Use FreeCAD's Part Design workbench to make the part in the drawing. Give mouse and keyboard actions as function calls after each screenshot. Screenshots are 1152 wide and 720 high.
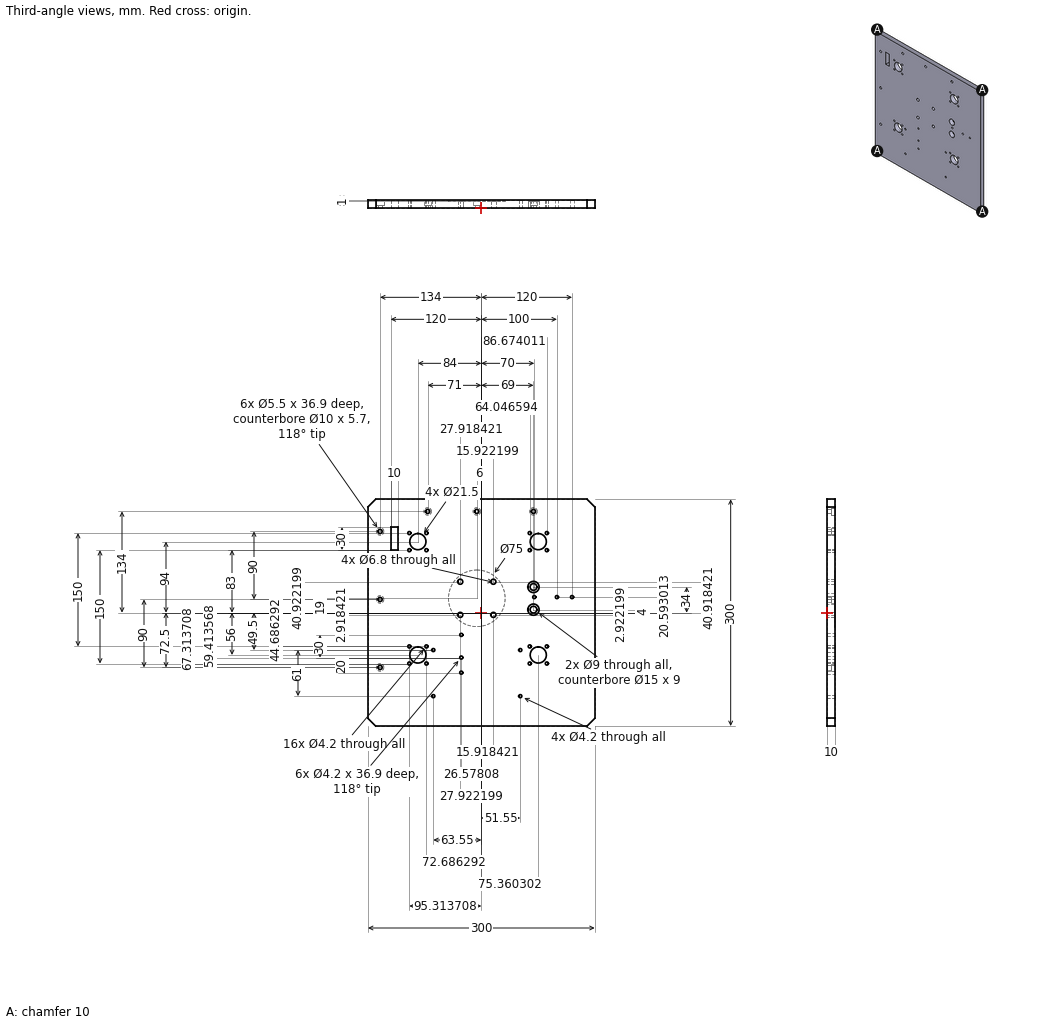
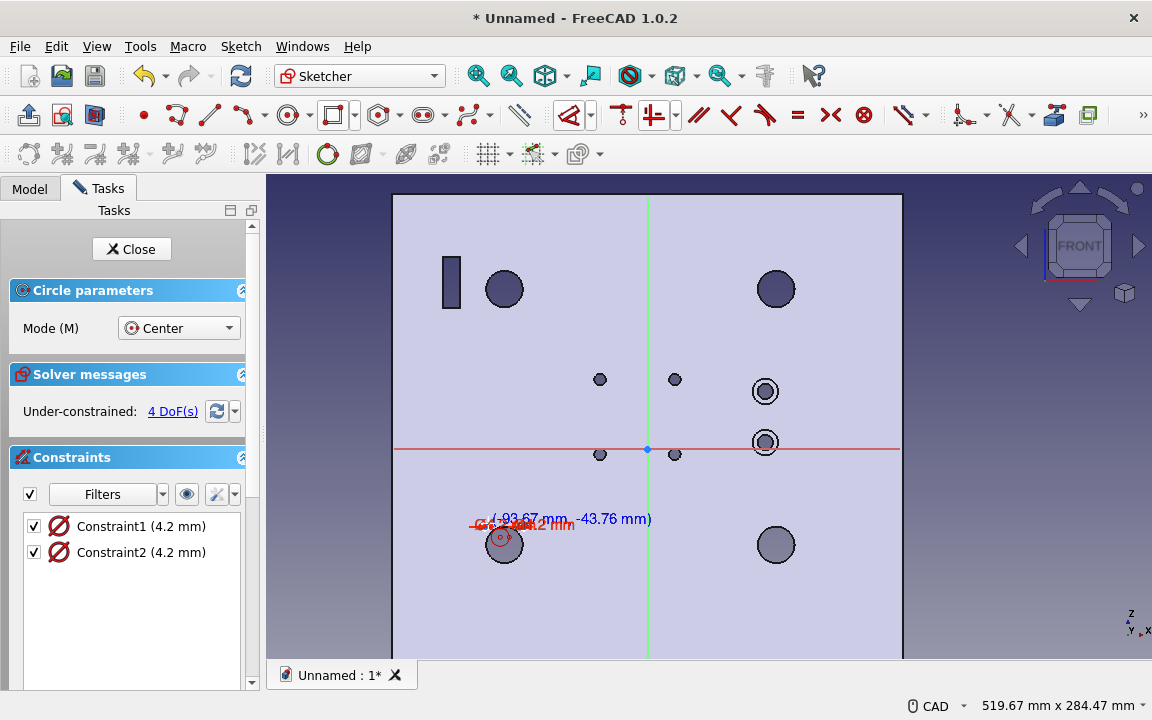
scroll(485, 564, up, 10)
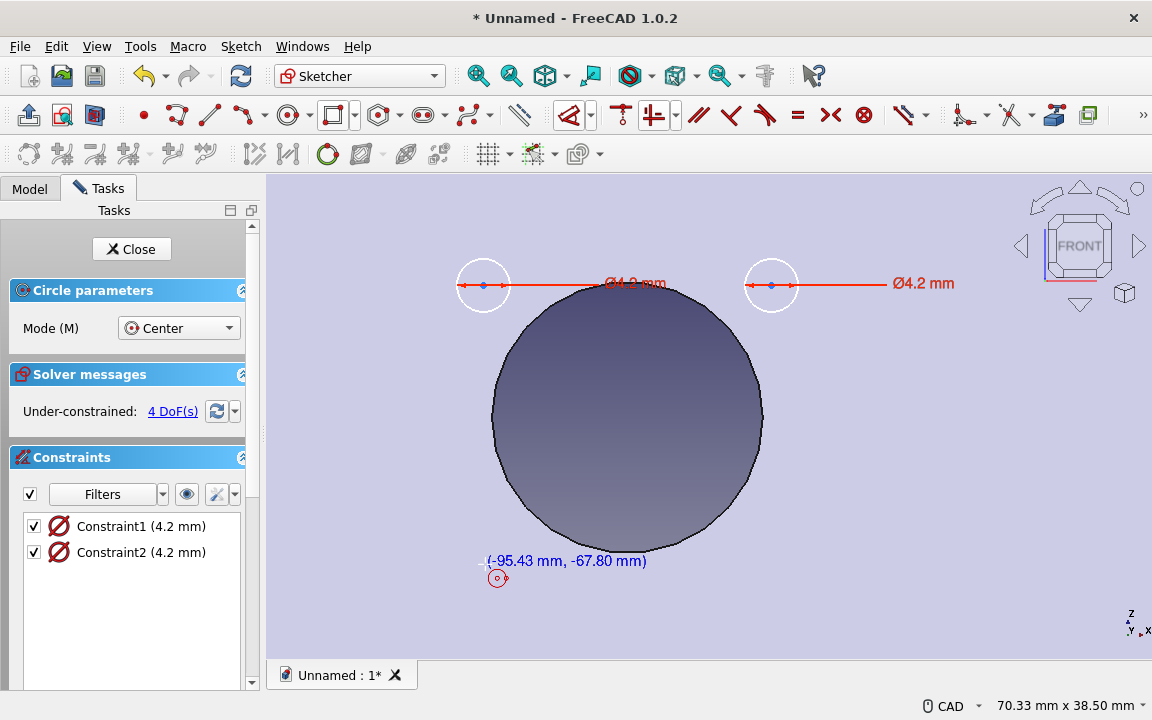
scroll(485, 564, down, 10)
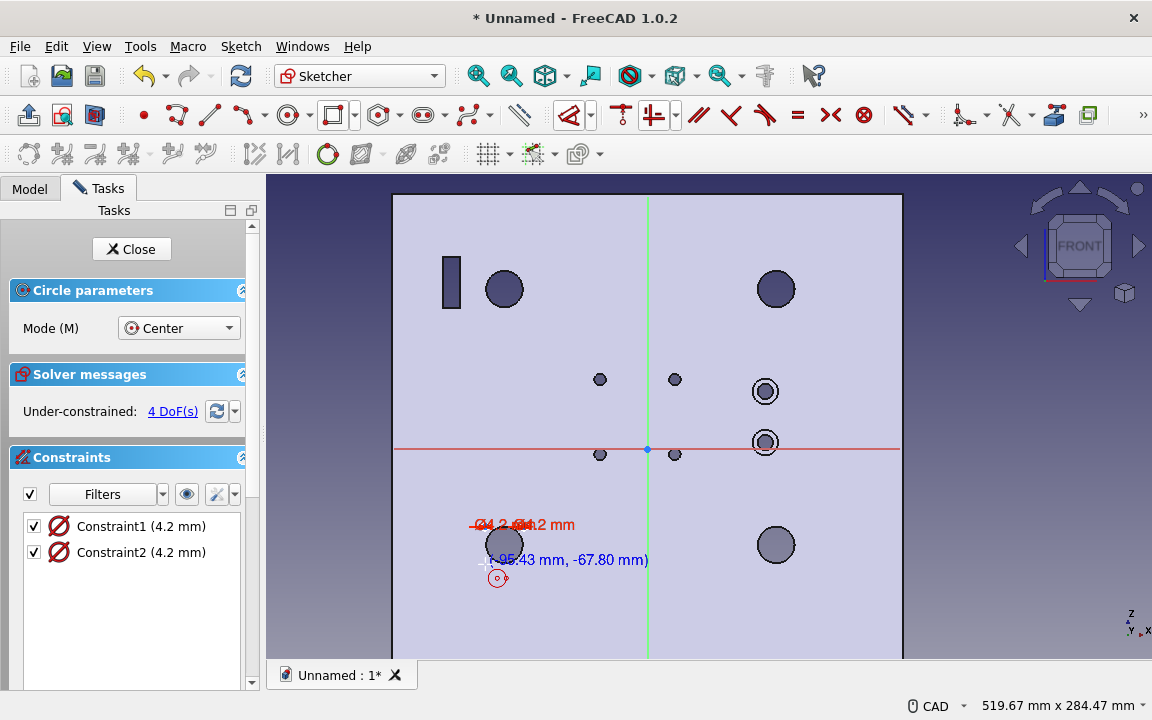
click(485, 564)
move(488, 562)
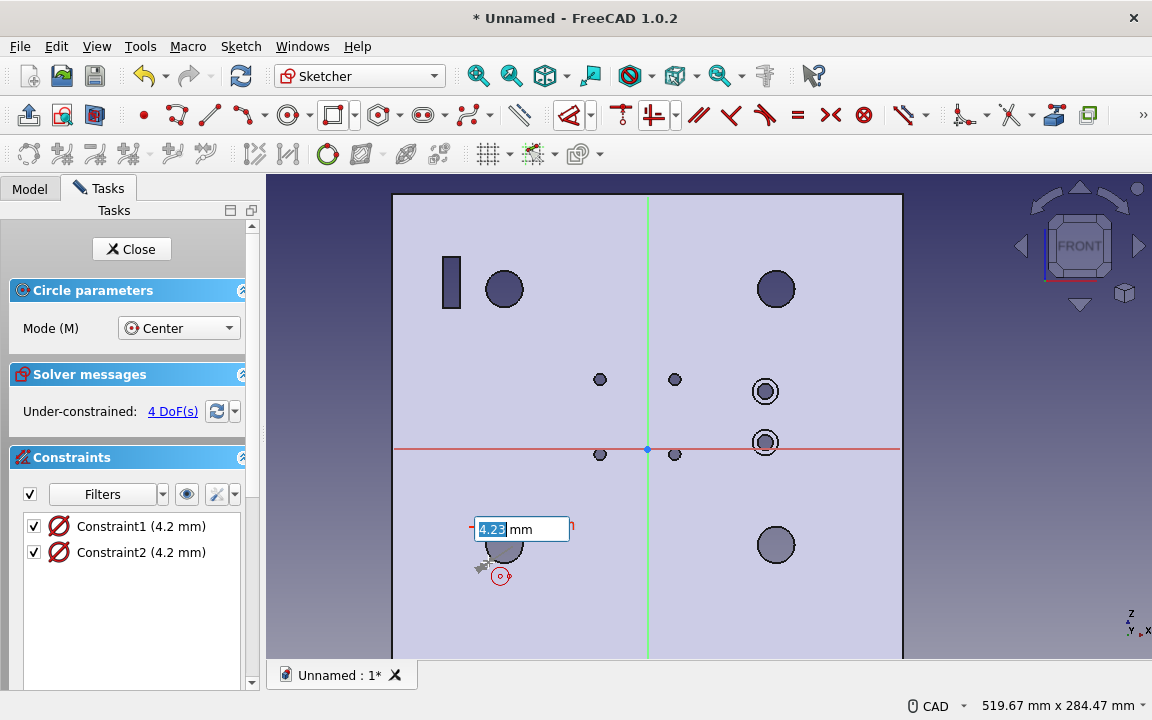
text(4.2)
key(Return)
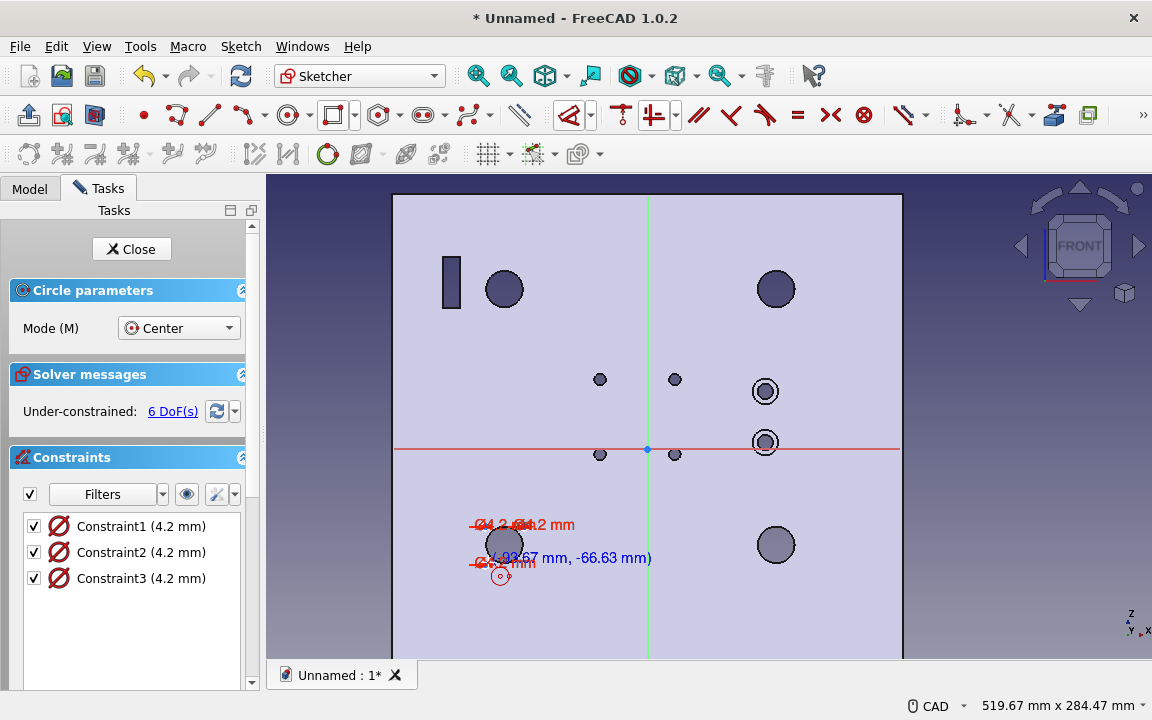
scroll(524, 564, up, 10)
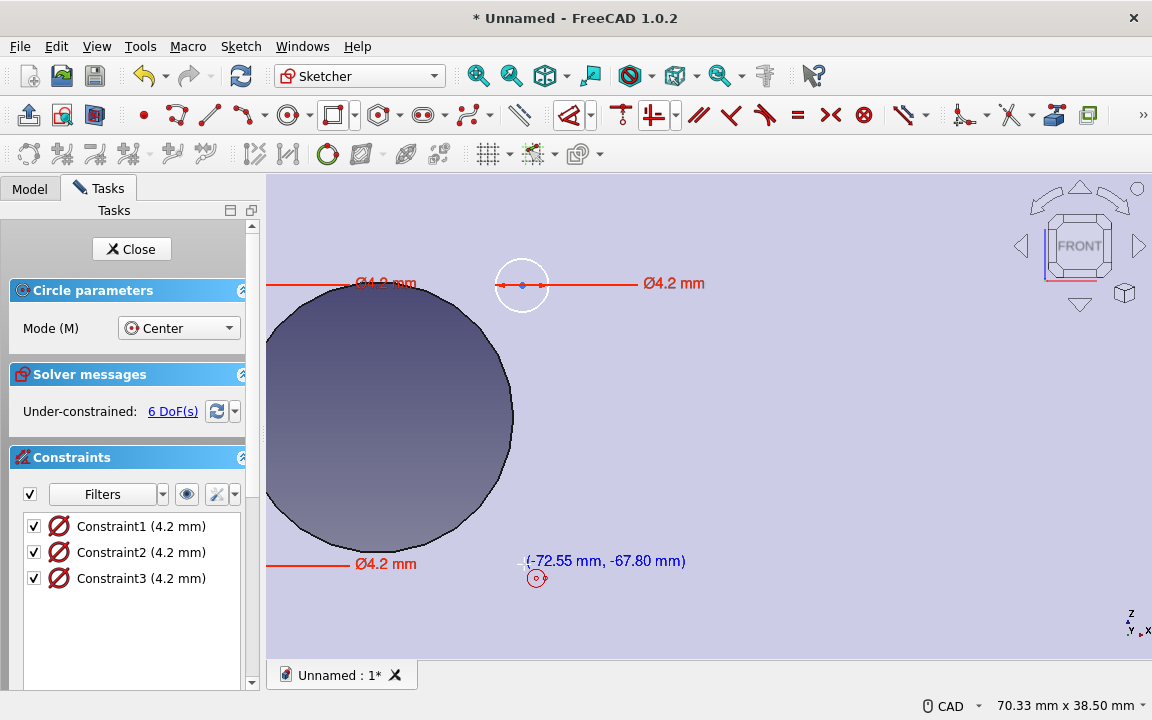
scroll(524, 564, down, 10)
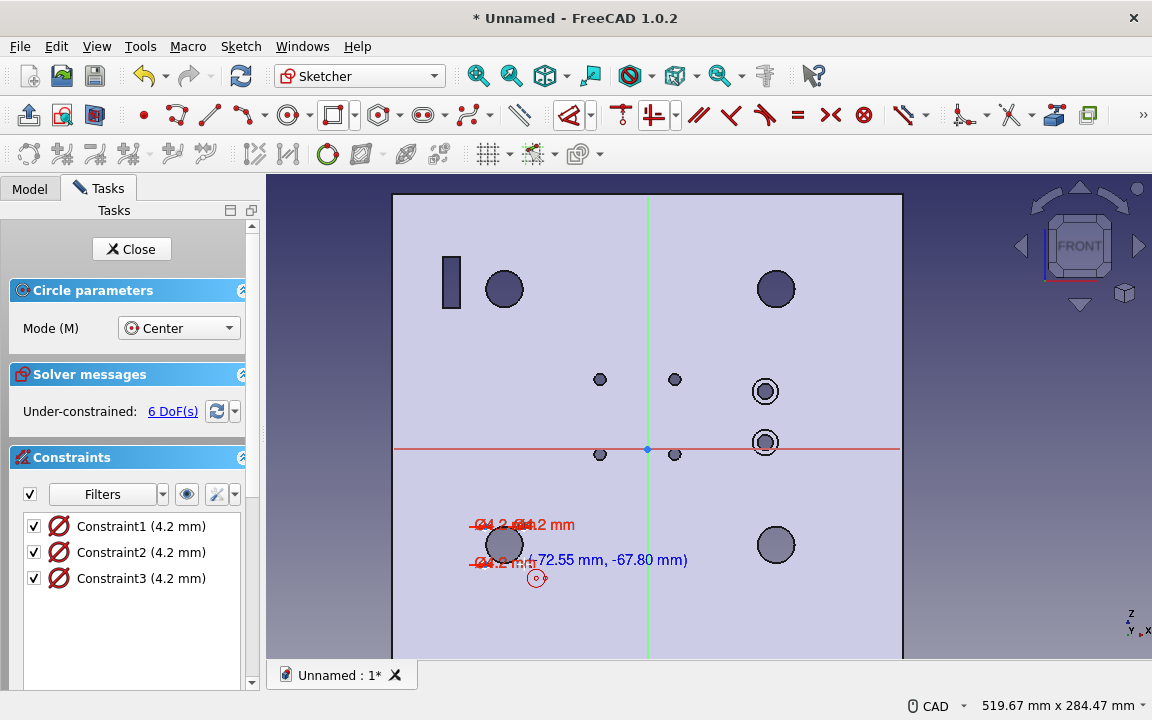
click(524, 564)
move(526, 562)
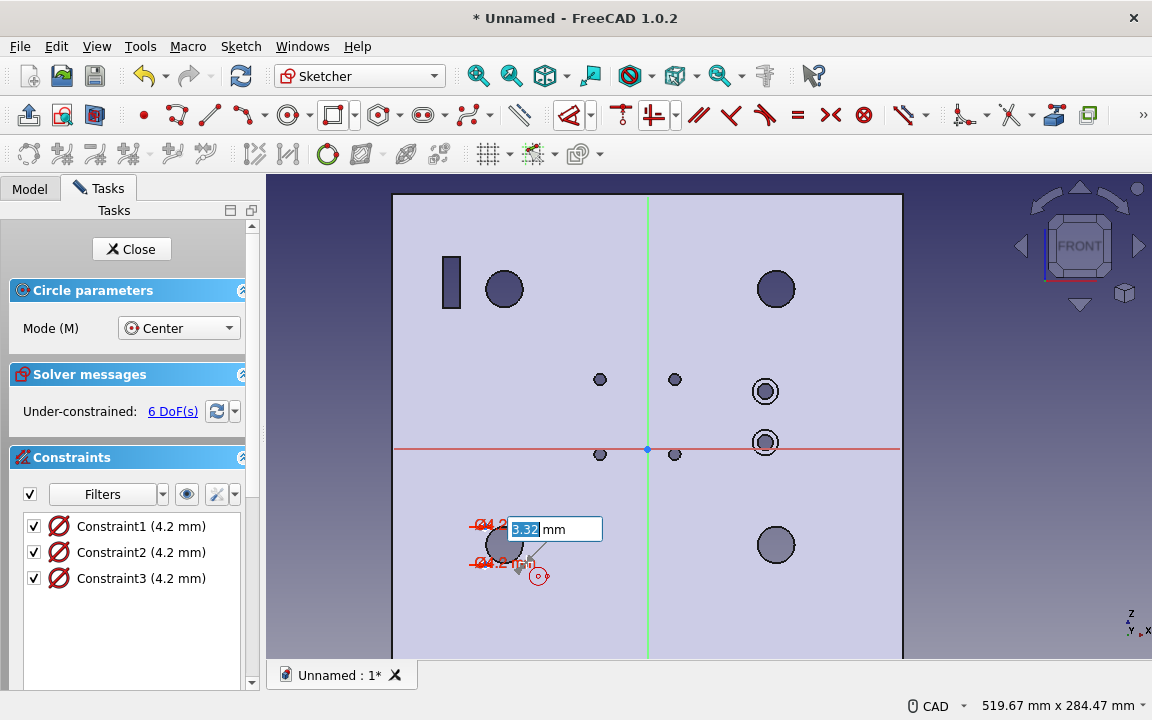
text(4.2)
key(Return)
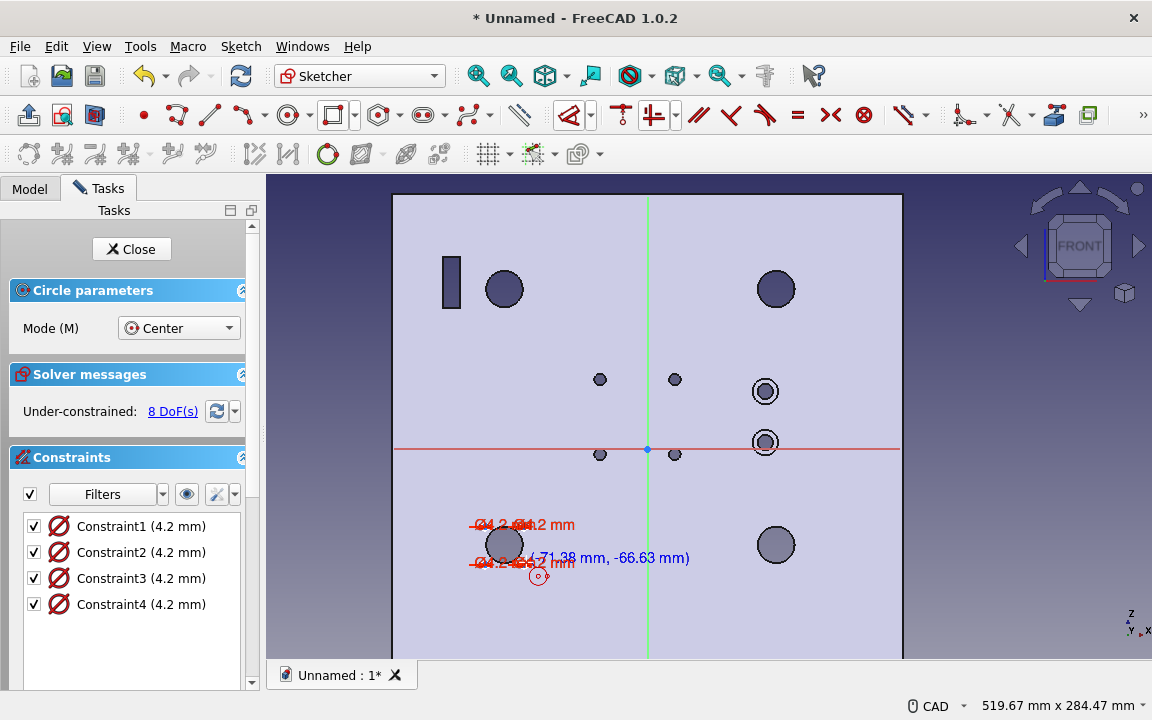
scroll(485, 308, up, 10)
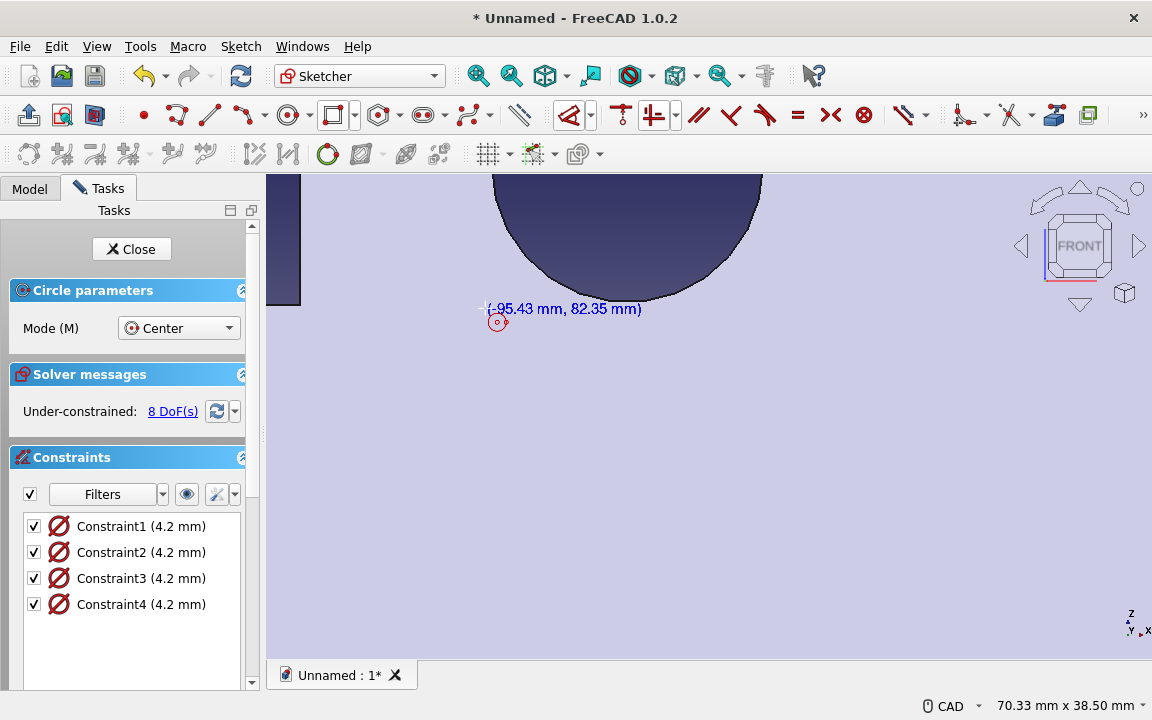
scroll(485, 308, down, 10)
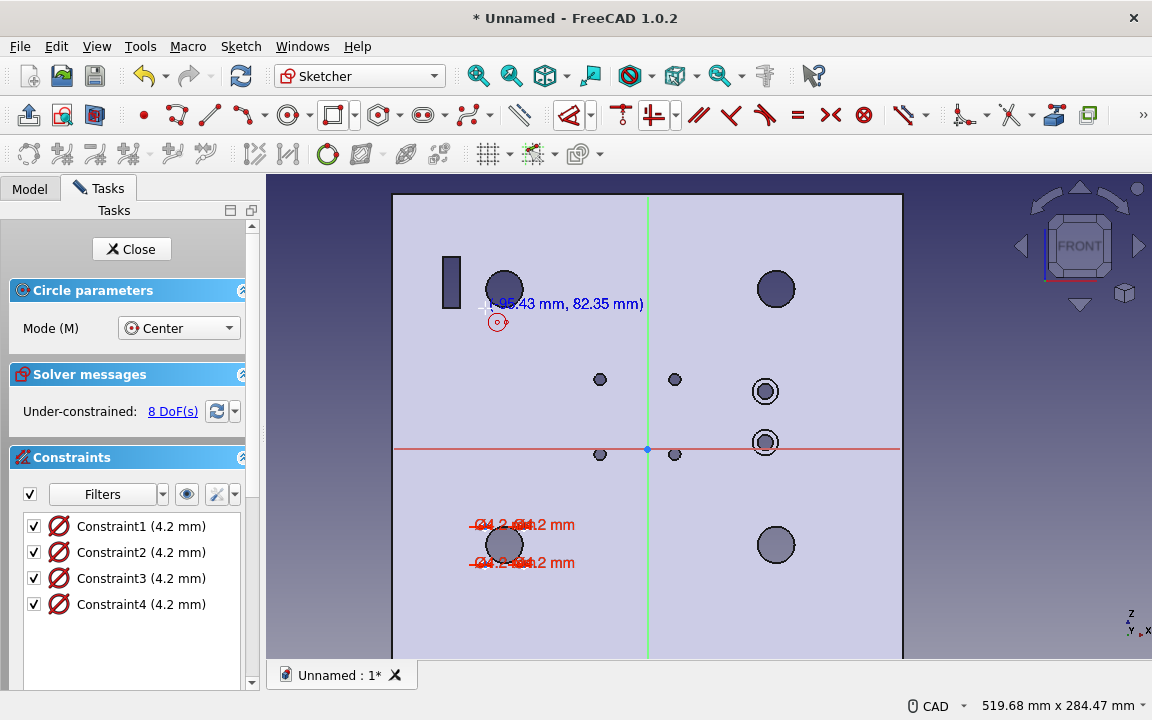
click(485, 308)
move(488, 306)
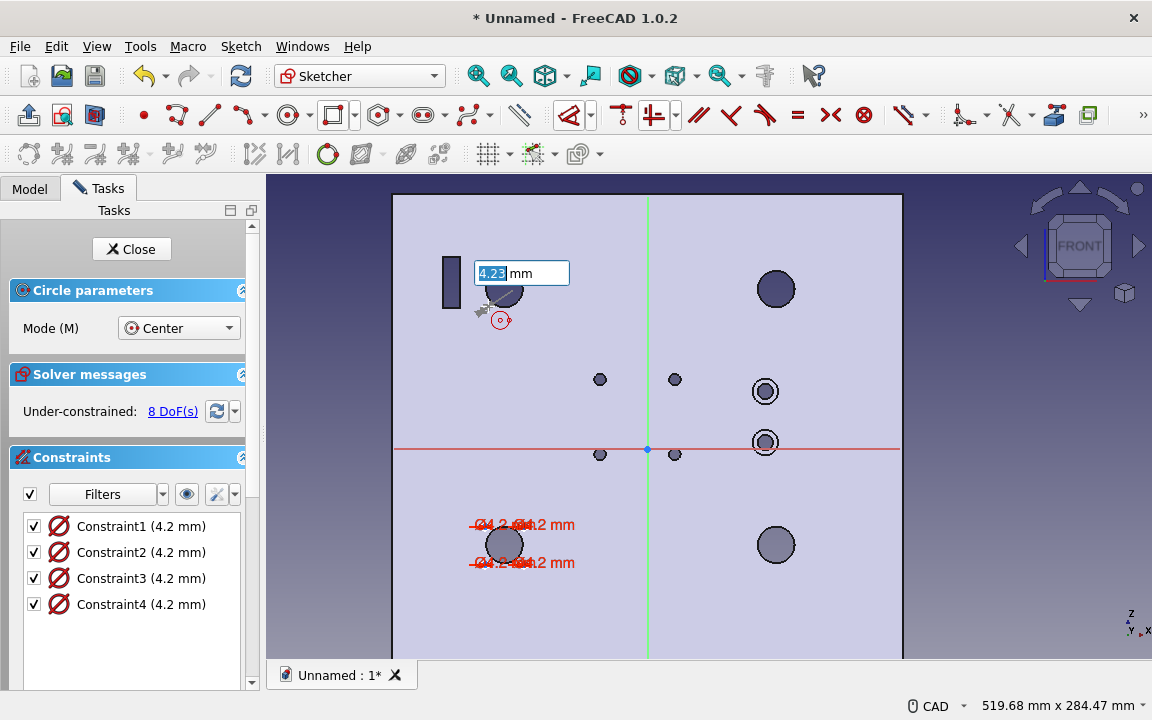
text(4.2)
key(Return)